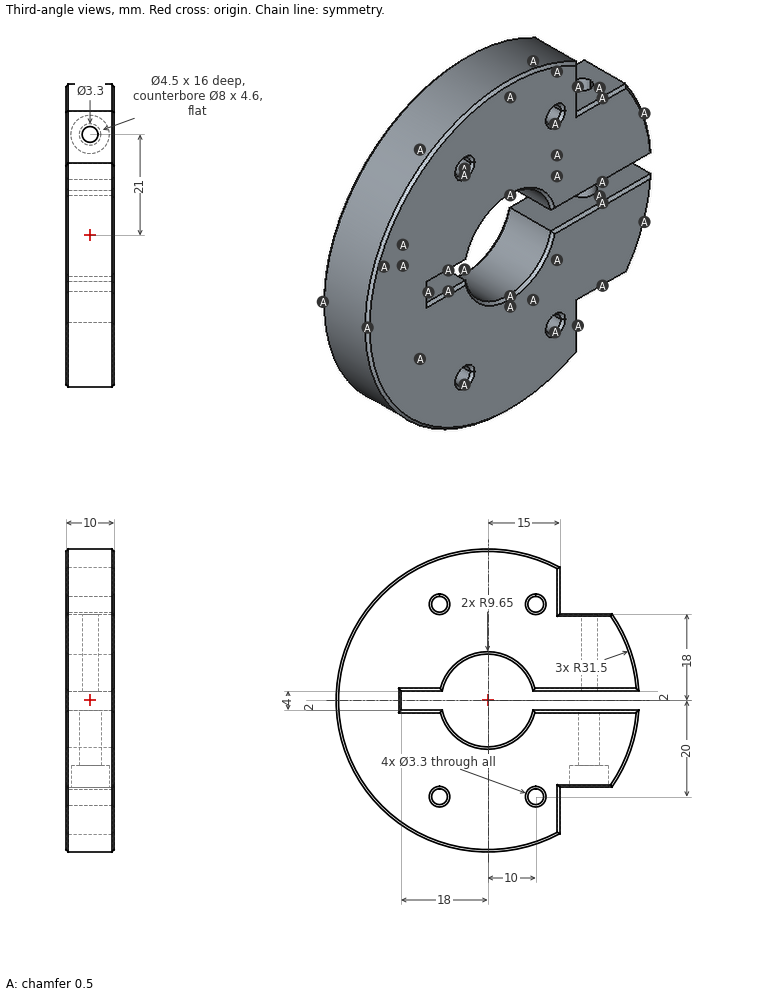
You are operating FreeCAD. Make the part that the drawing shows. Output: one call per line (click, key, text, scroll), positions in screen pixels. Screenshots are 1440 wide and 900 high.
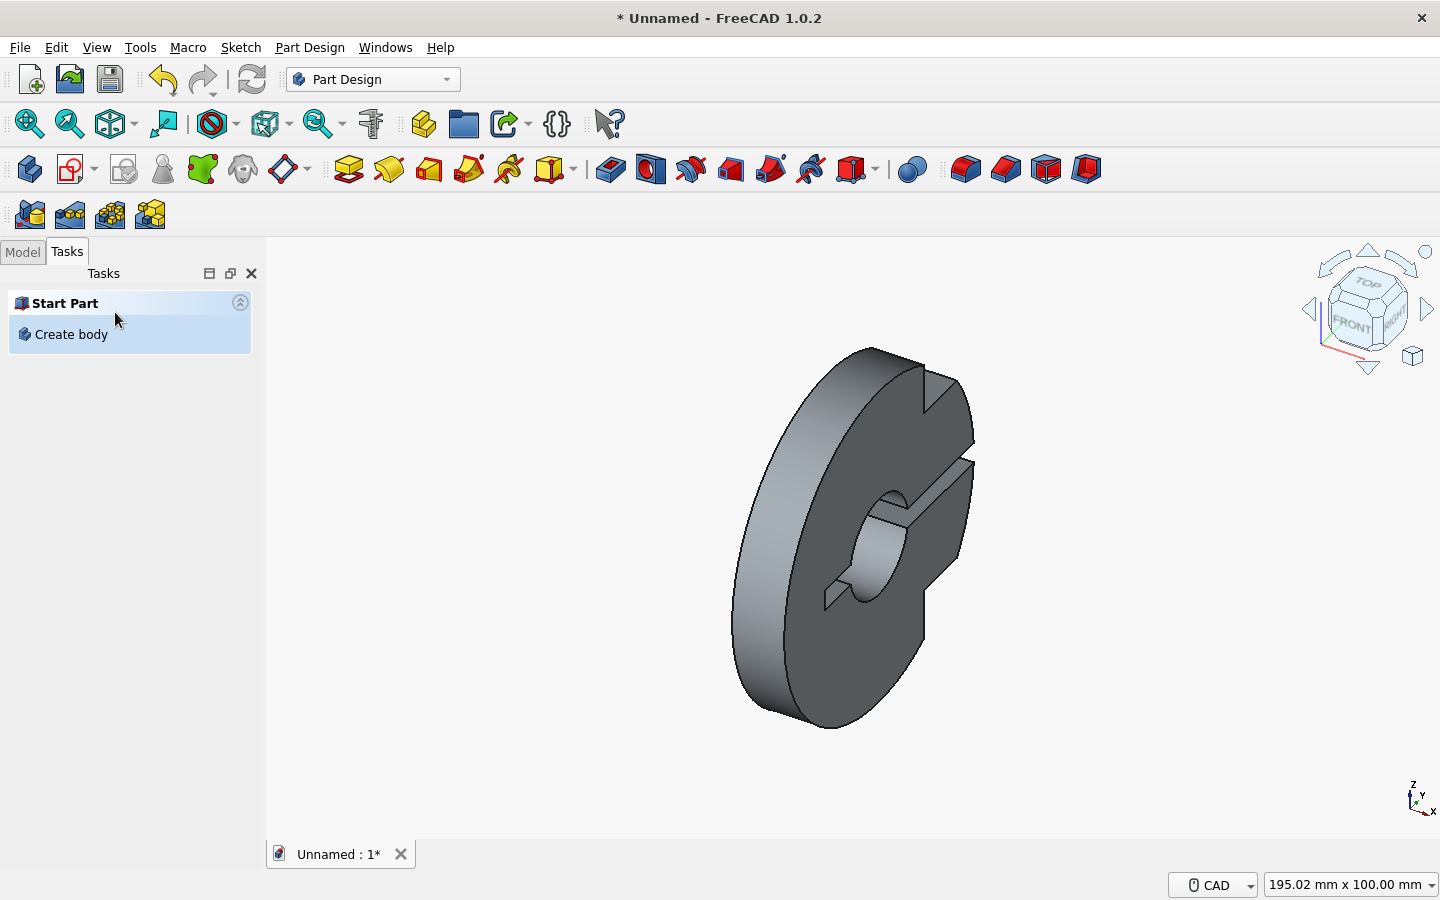
key(5)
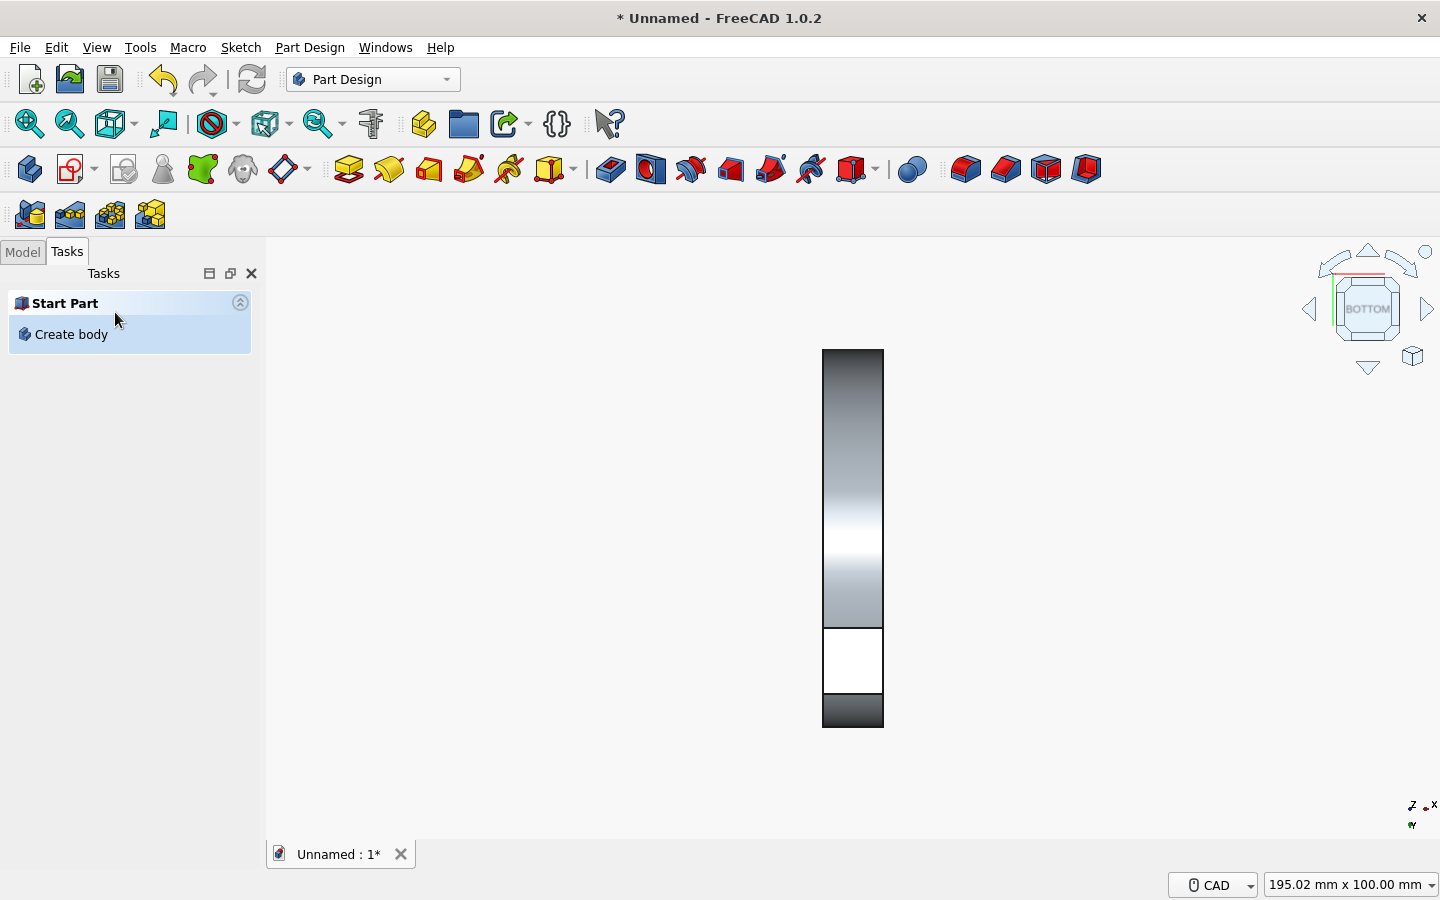
click(853, 660)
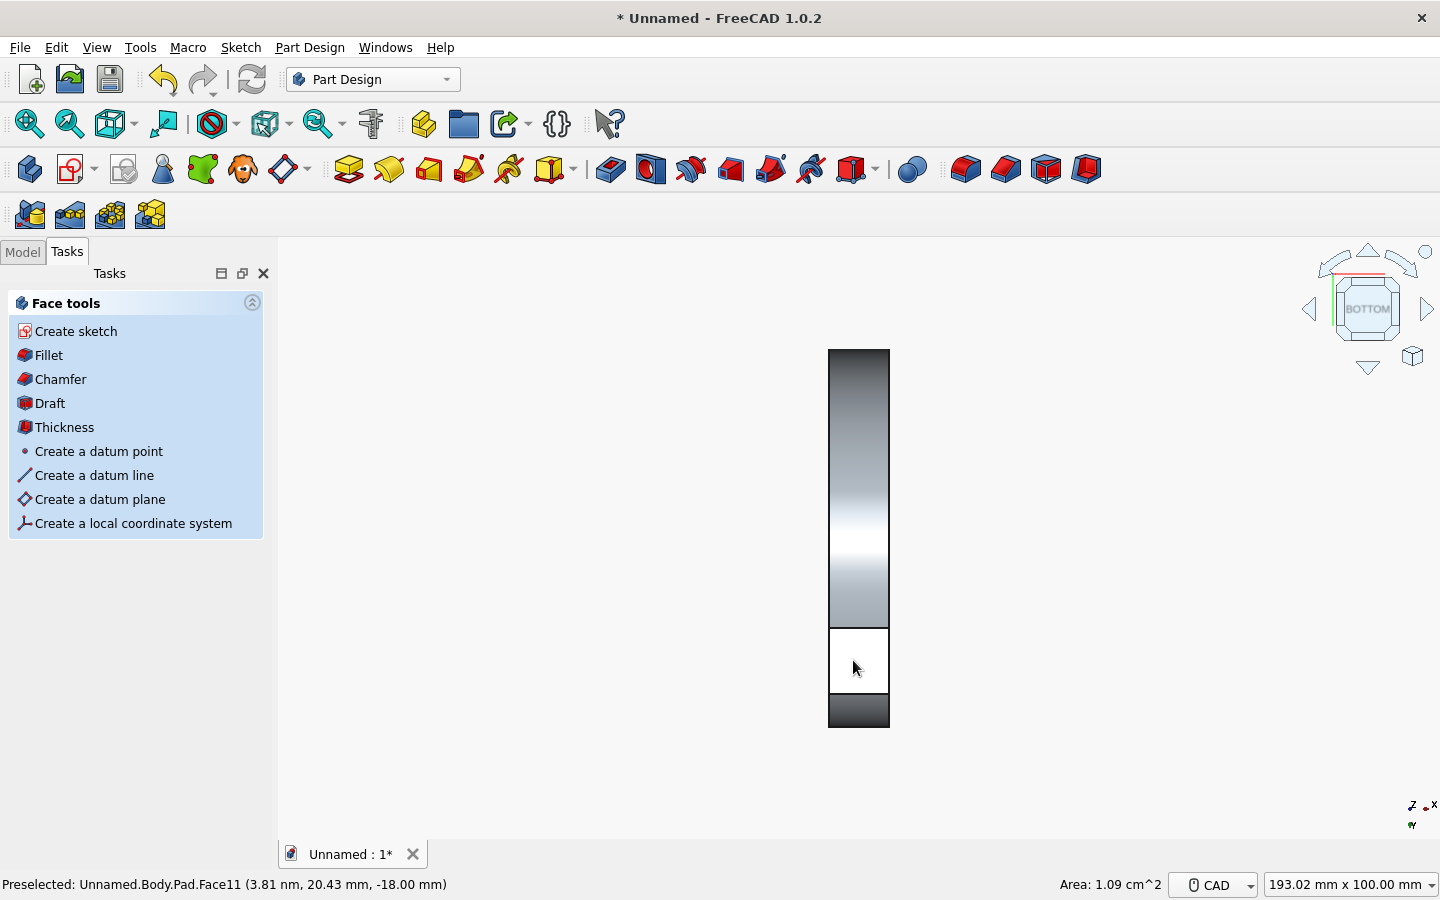
click(70, 170)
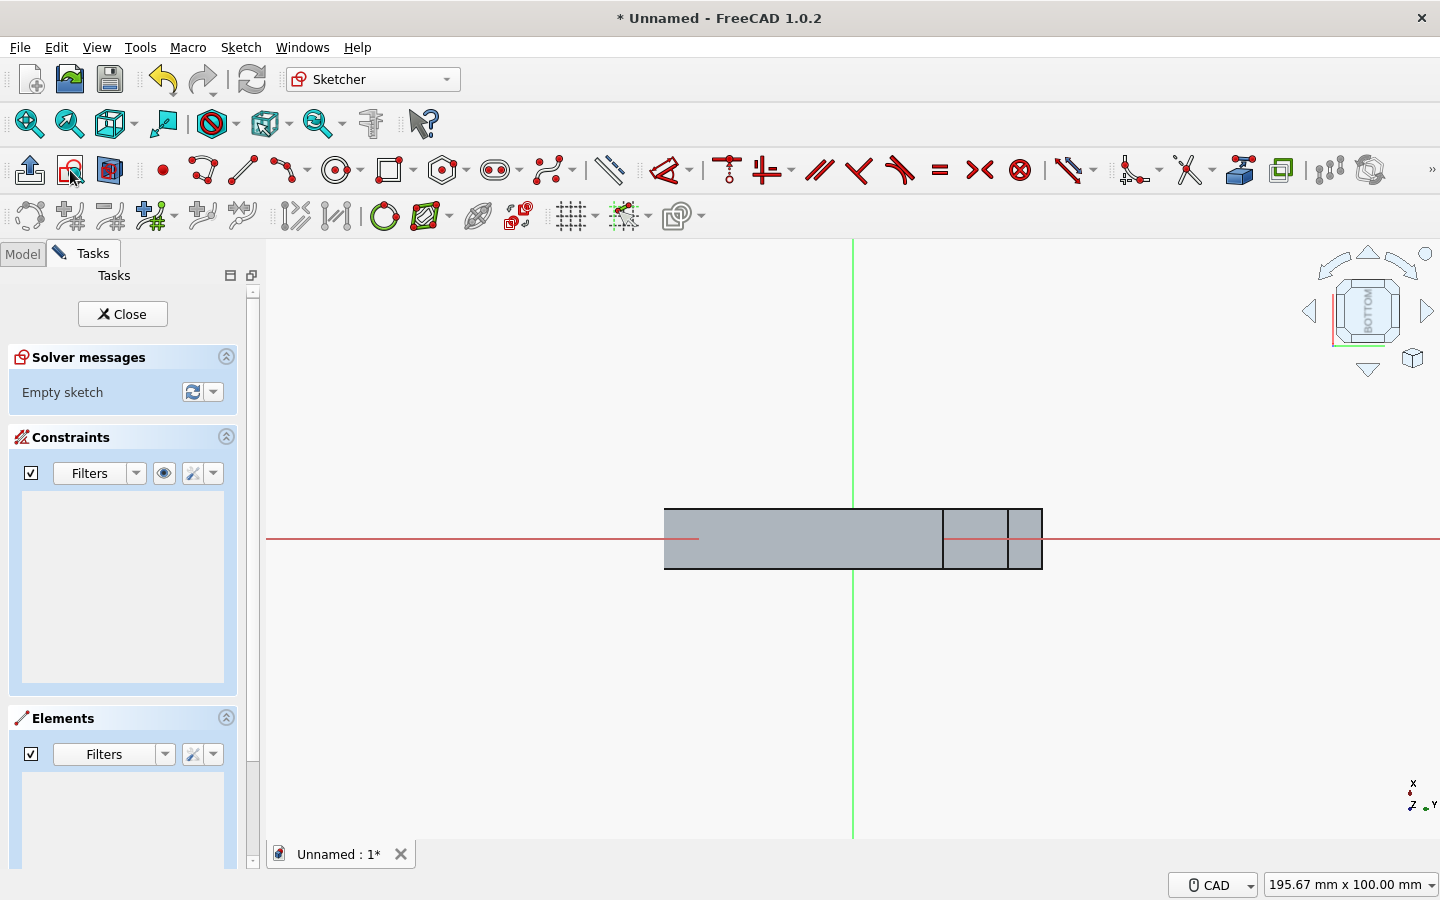
click(110, 170)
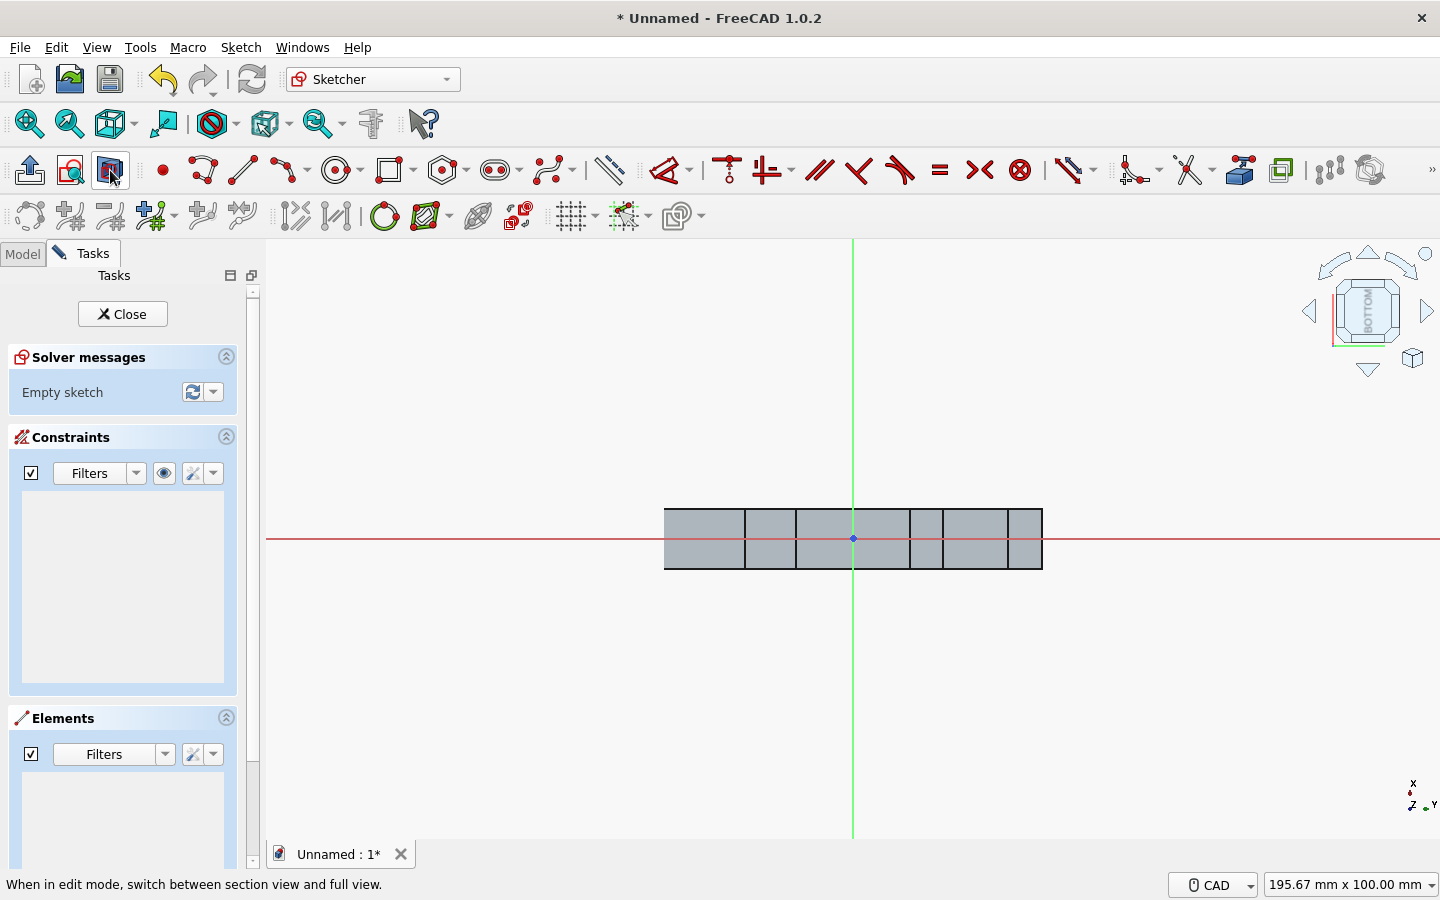
scroll(995, 539, up, 13)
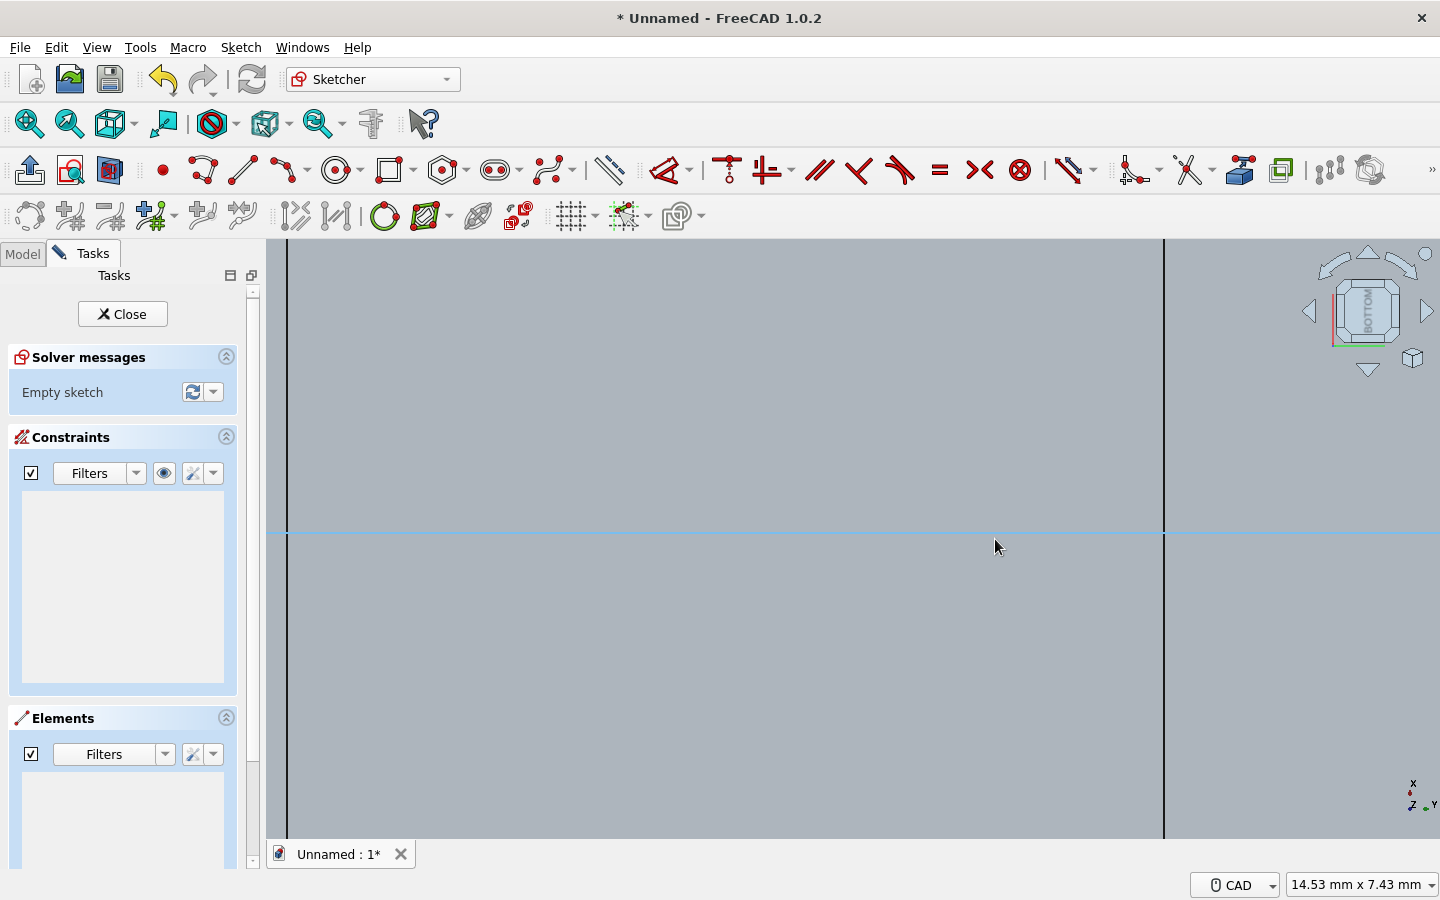
key(g)
key(c)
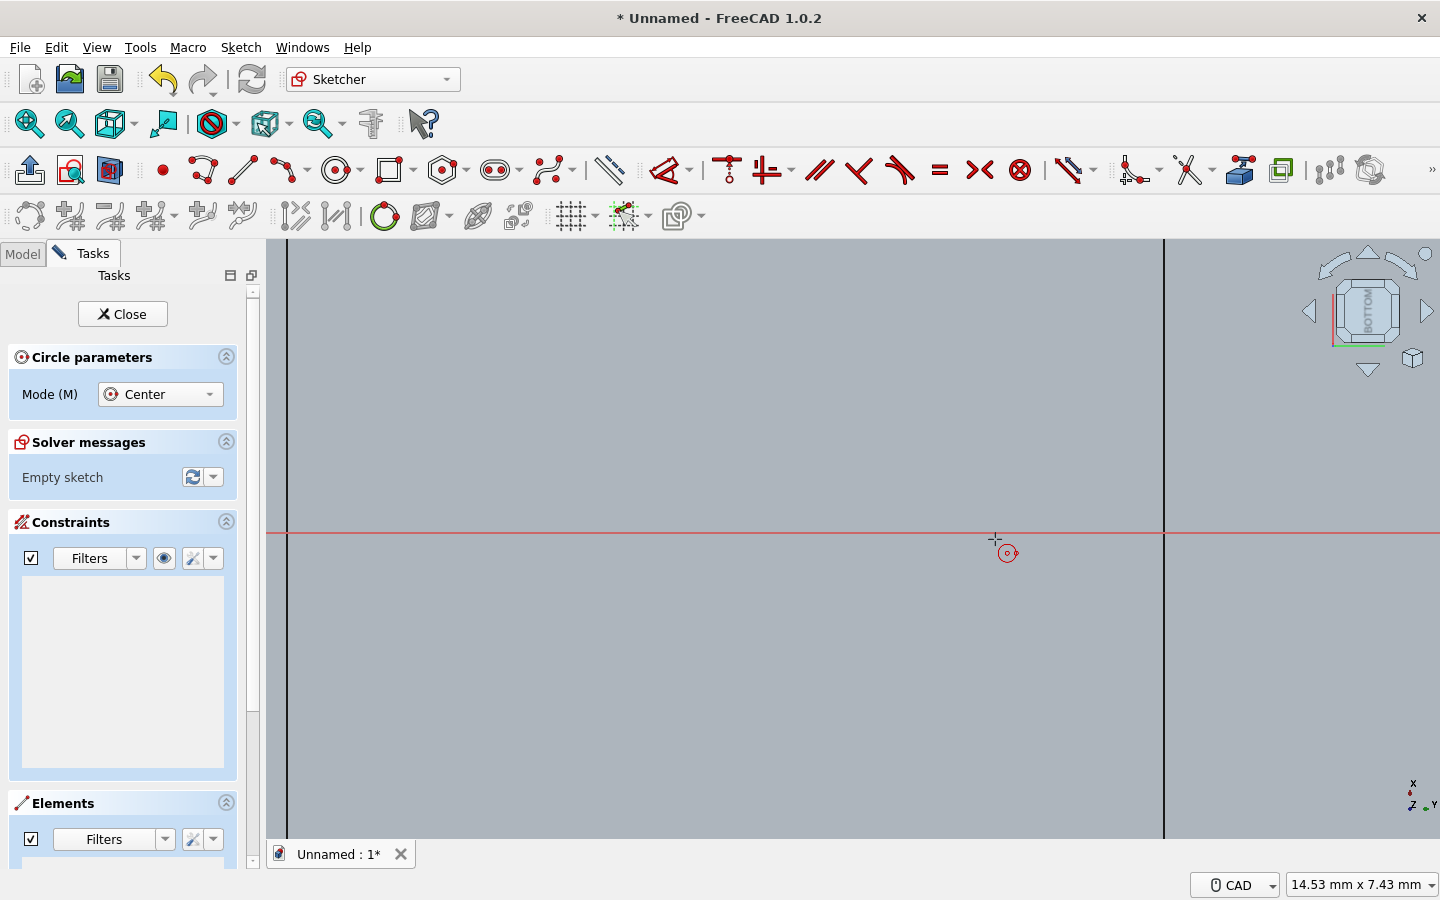
click(772, 533)
click(900, 404)
key(Escape)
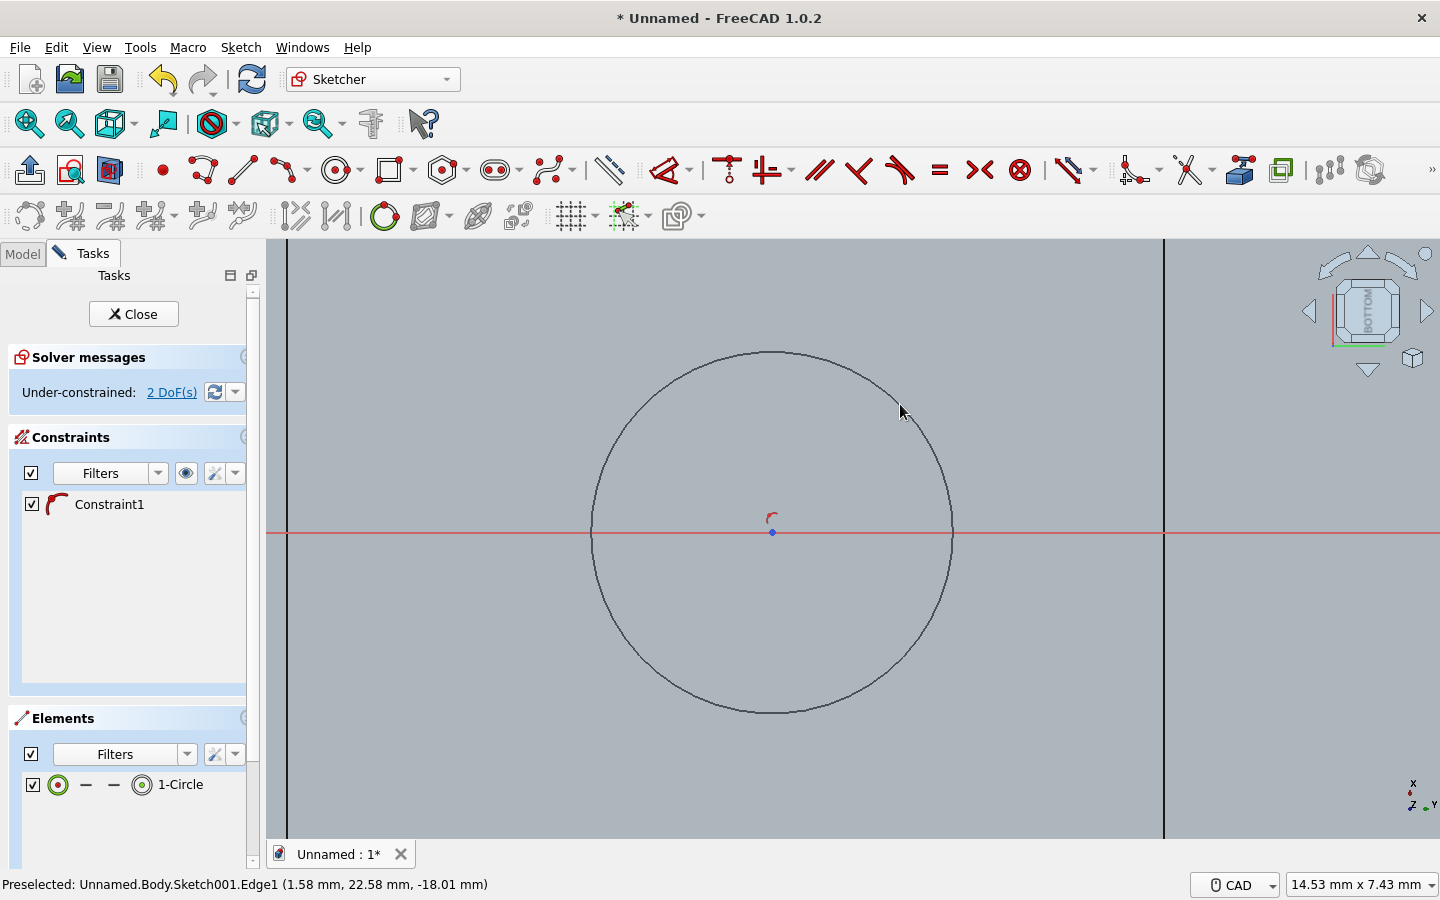
key(d)